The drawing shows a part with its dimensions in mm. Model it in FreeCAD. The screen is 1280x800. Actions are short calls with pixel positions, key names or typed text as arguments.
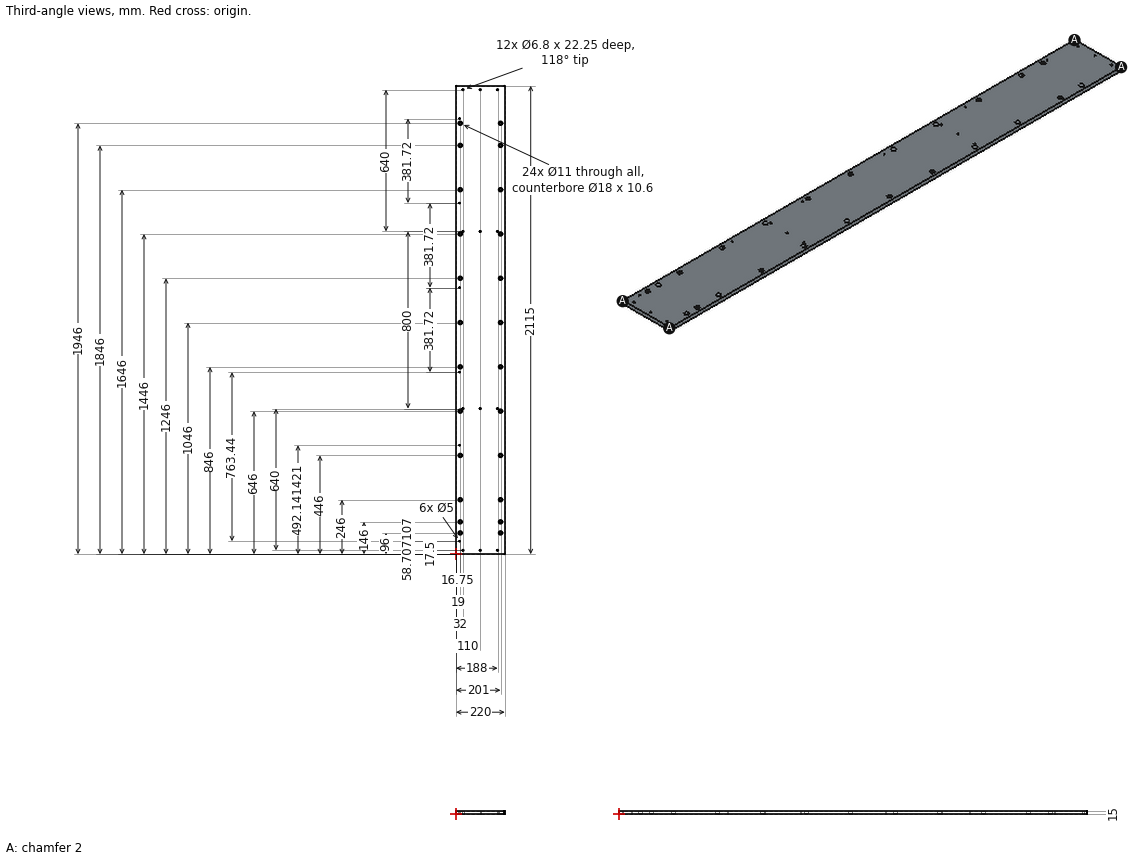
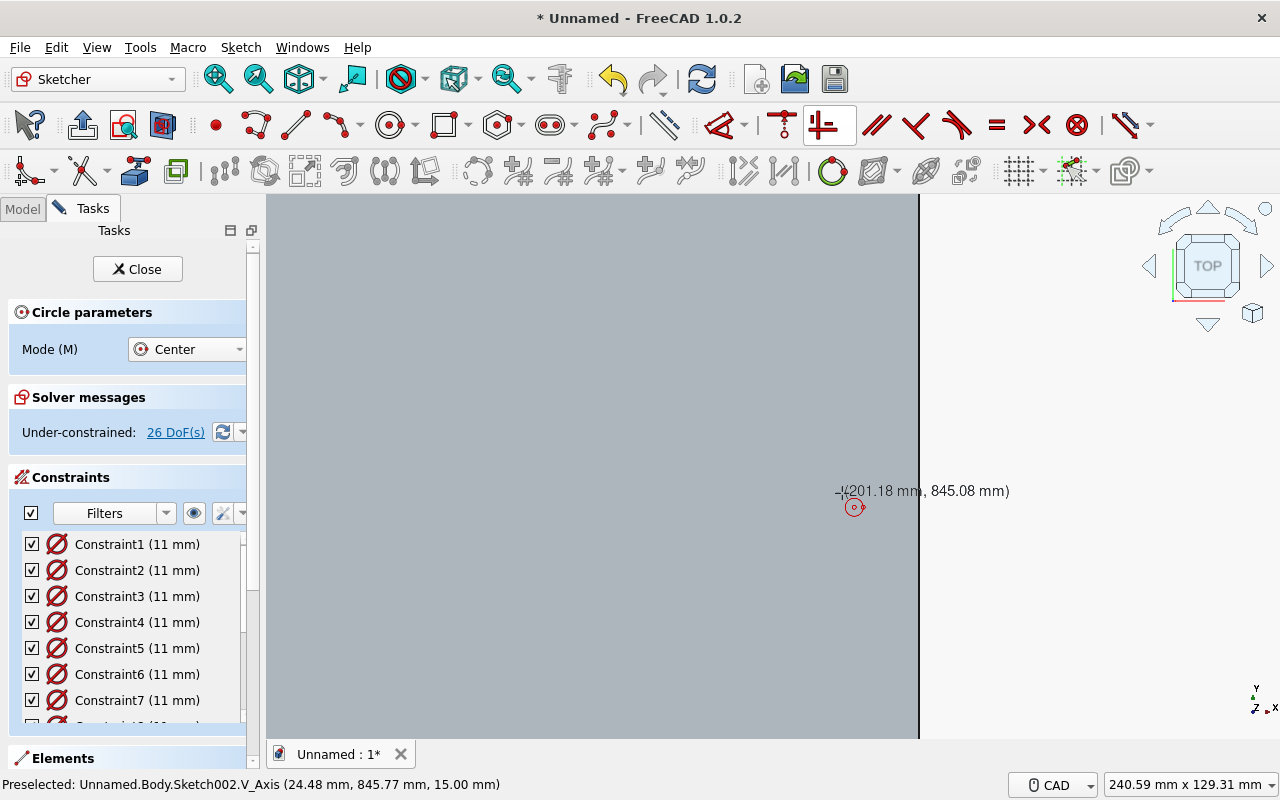
scroll(719, 494, down, 15)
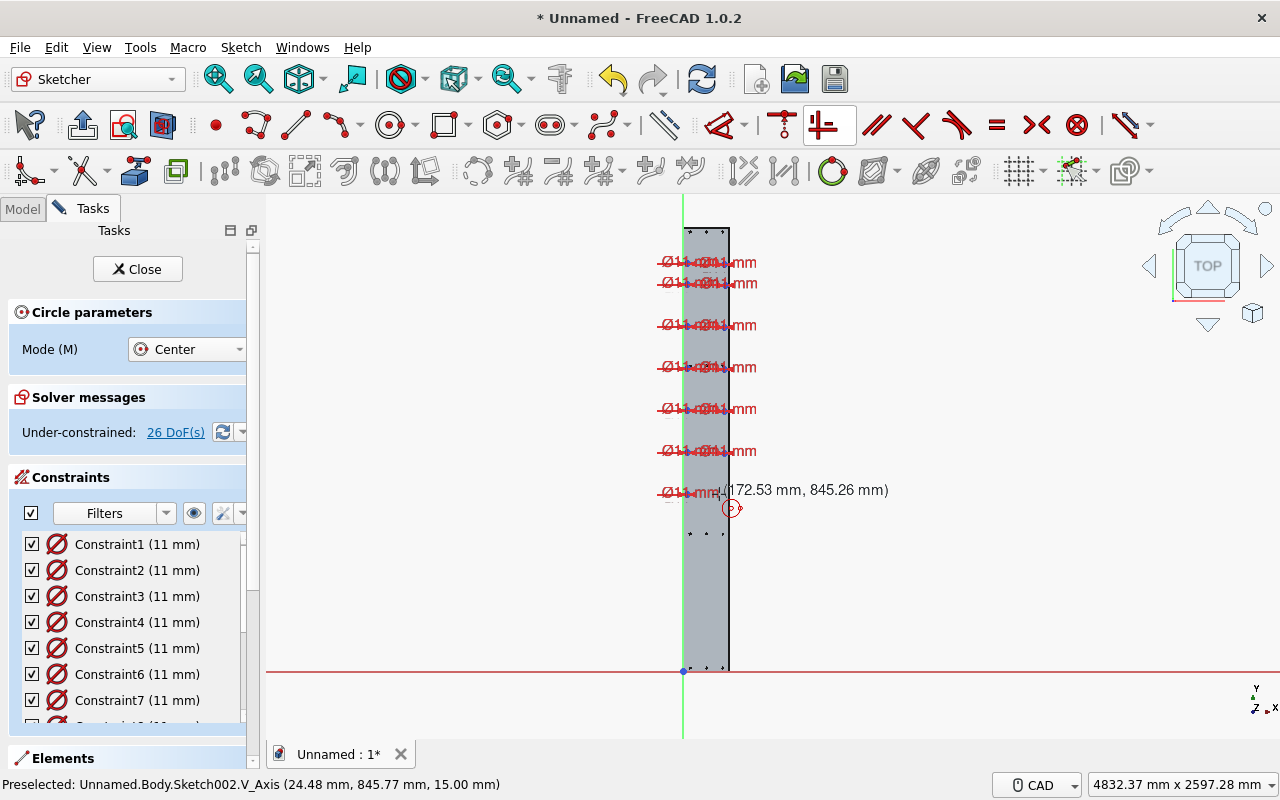
click(725, 494)
move(726, 494)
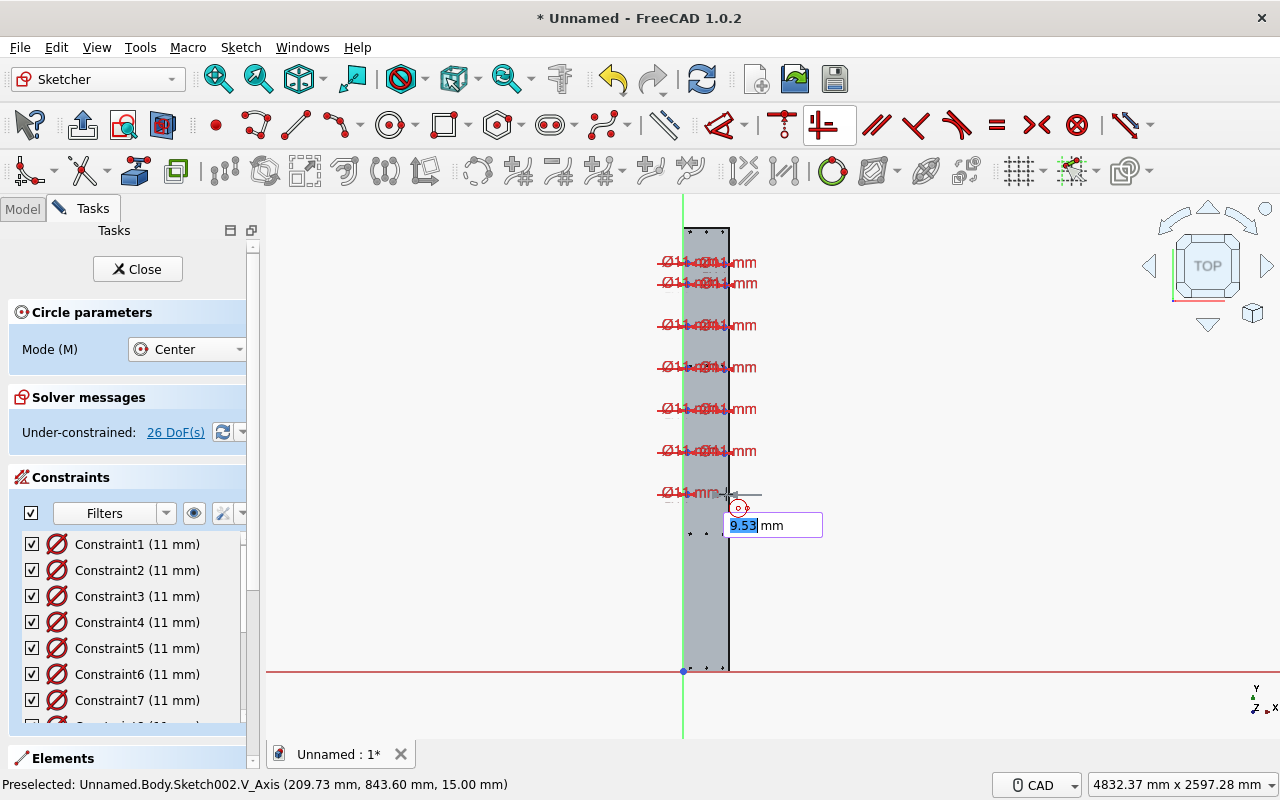
text(11)
key(Return)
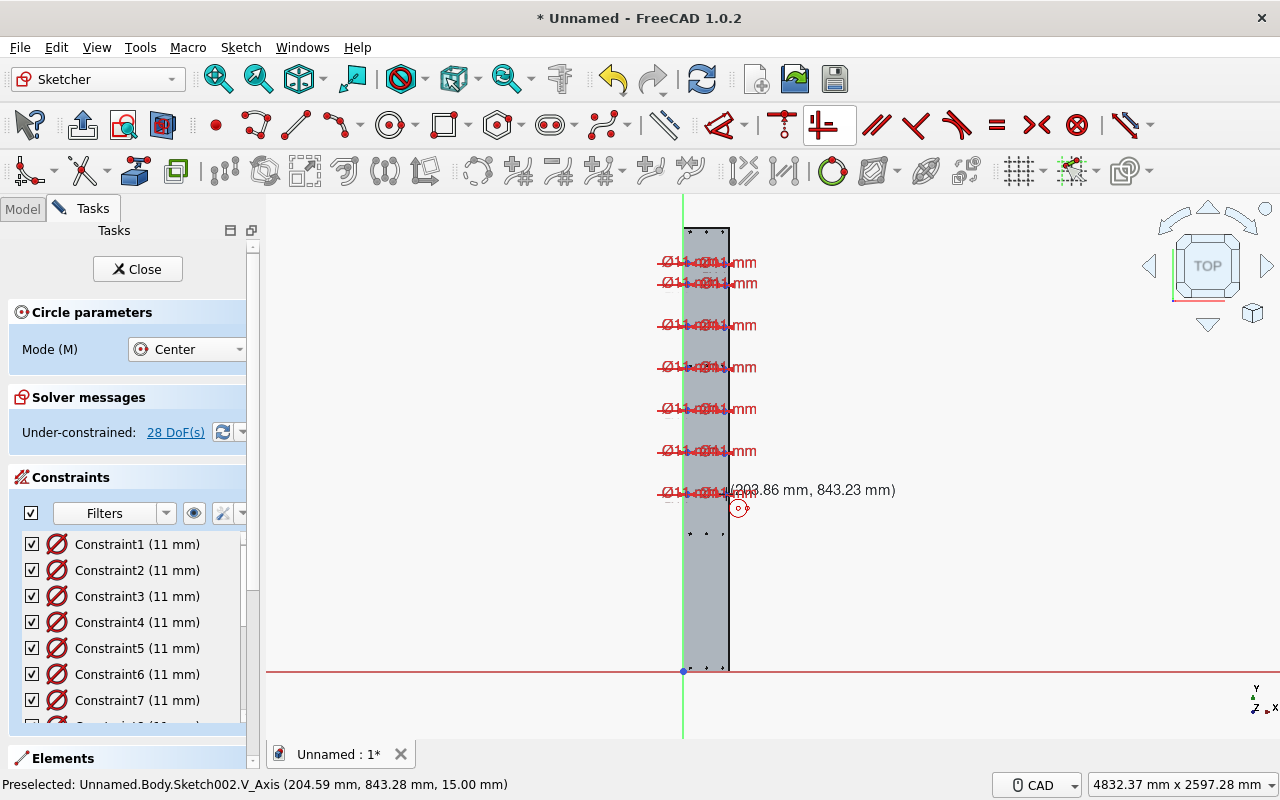
scroll(687, 536, up, 15)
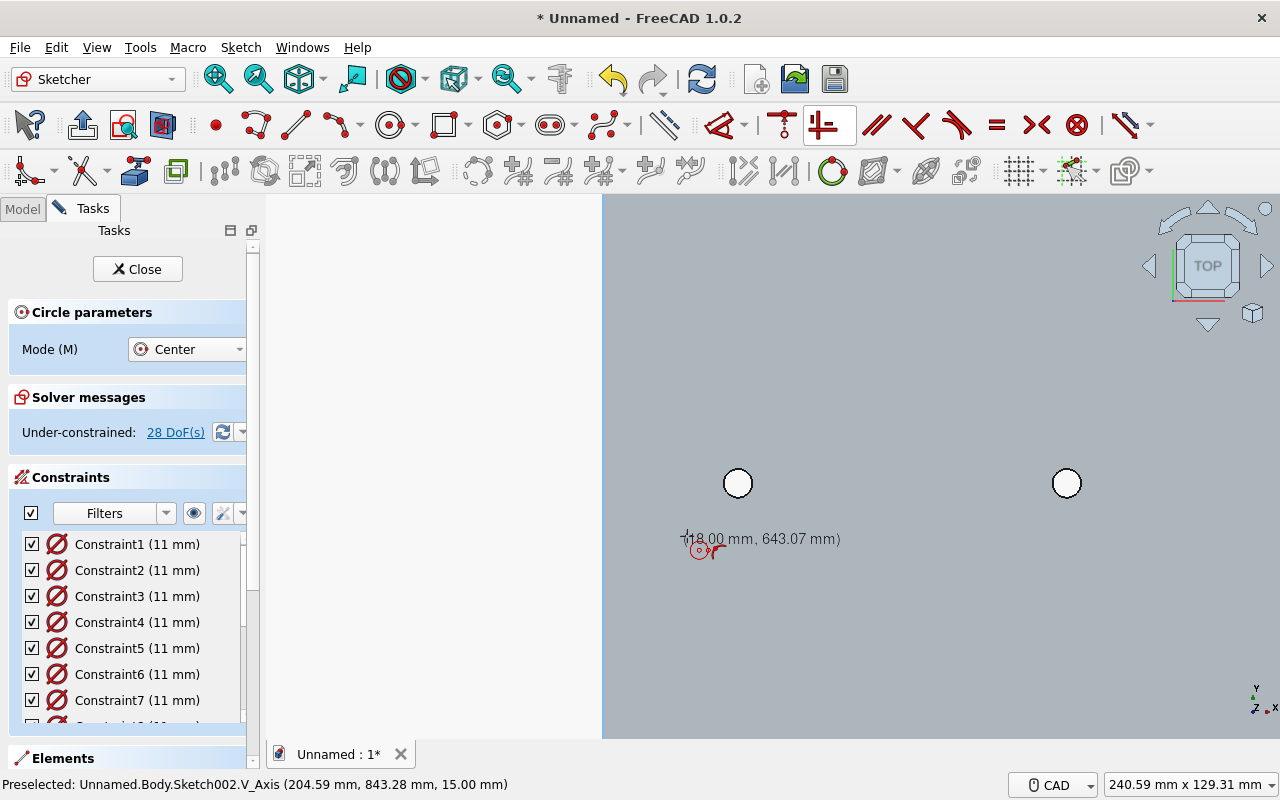
scroll(687, 536, down, 15)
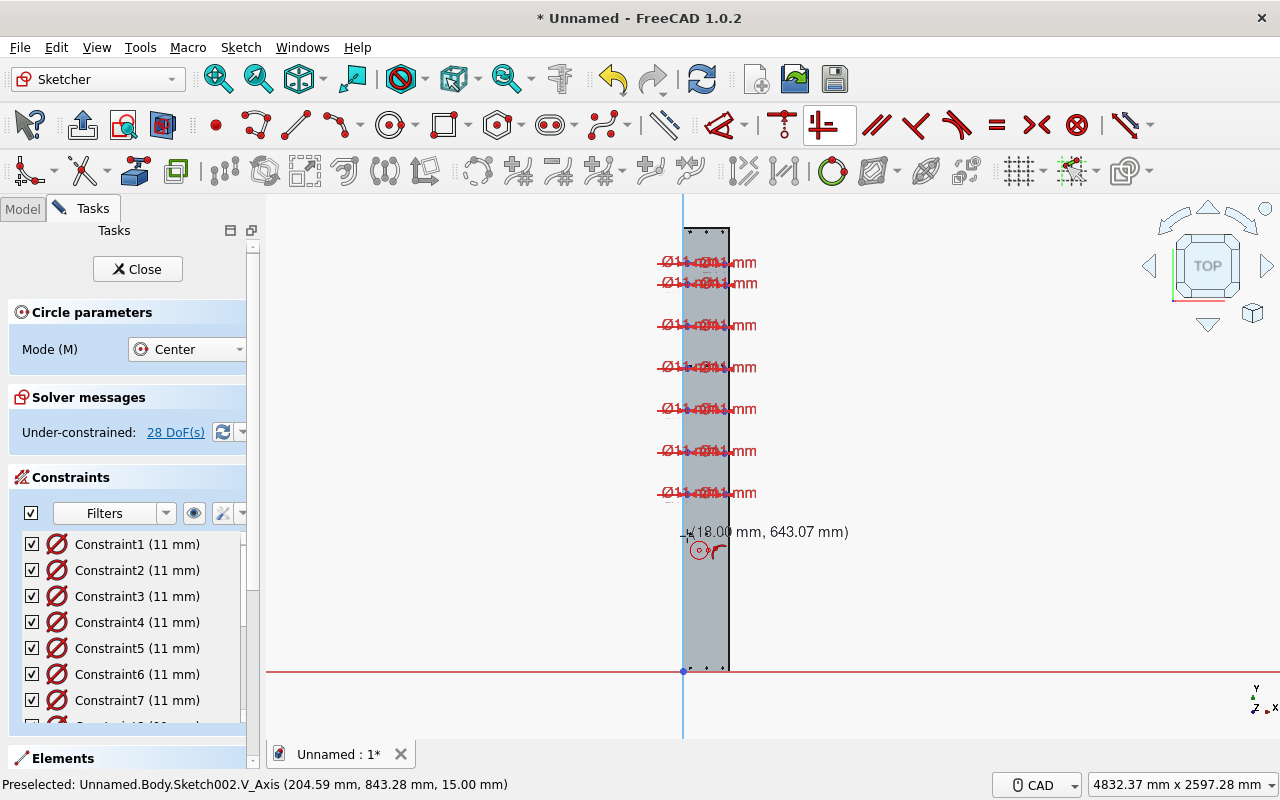
scroll(687, 536, up, 7)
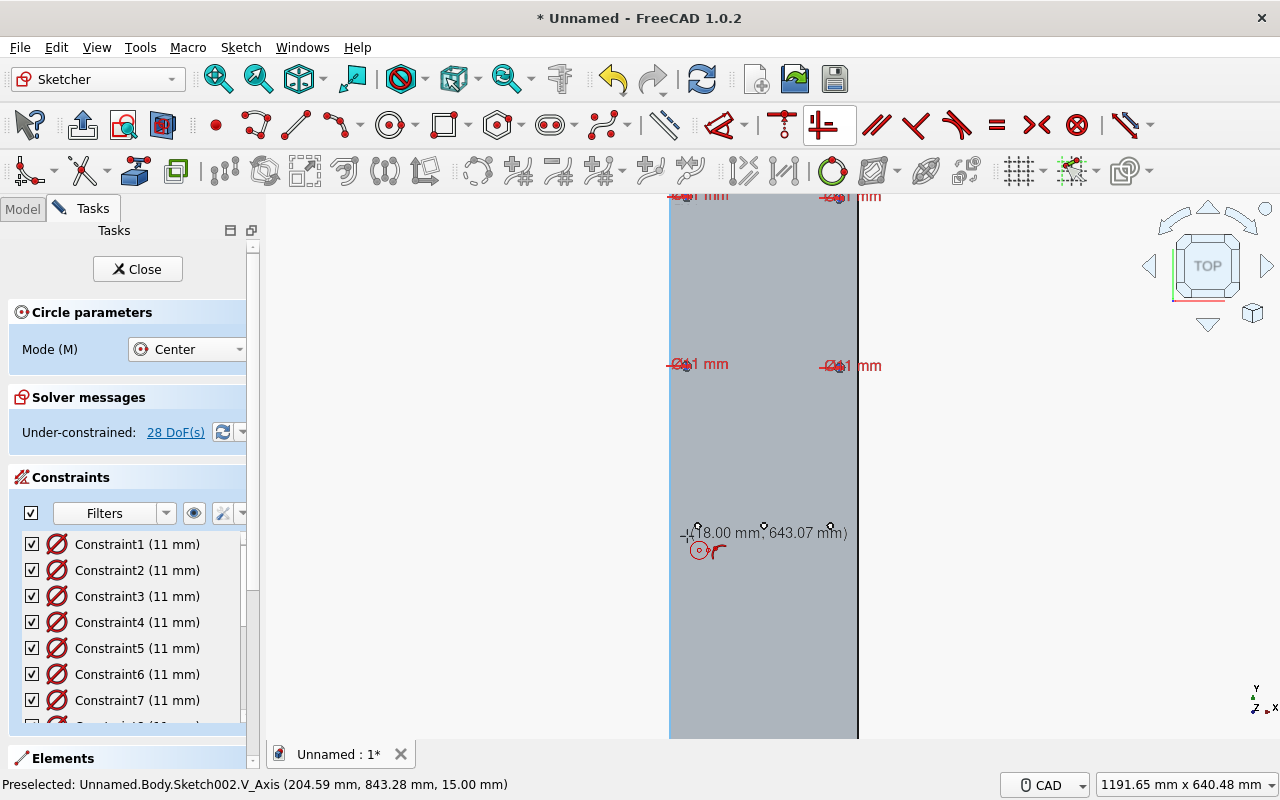
click(687, 536)
move(690, 532)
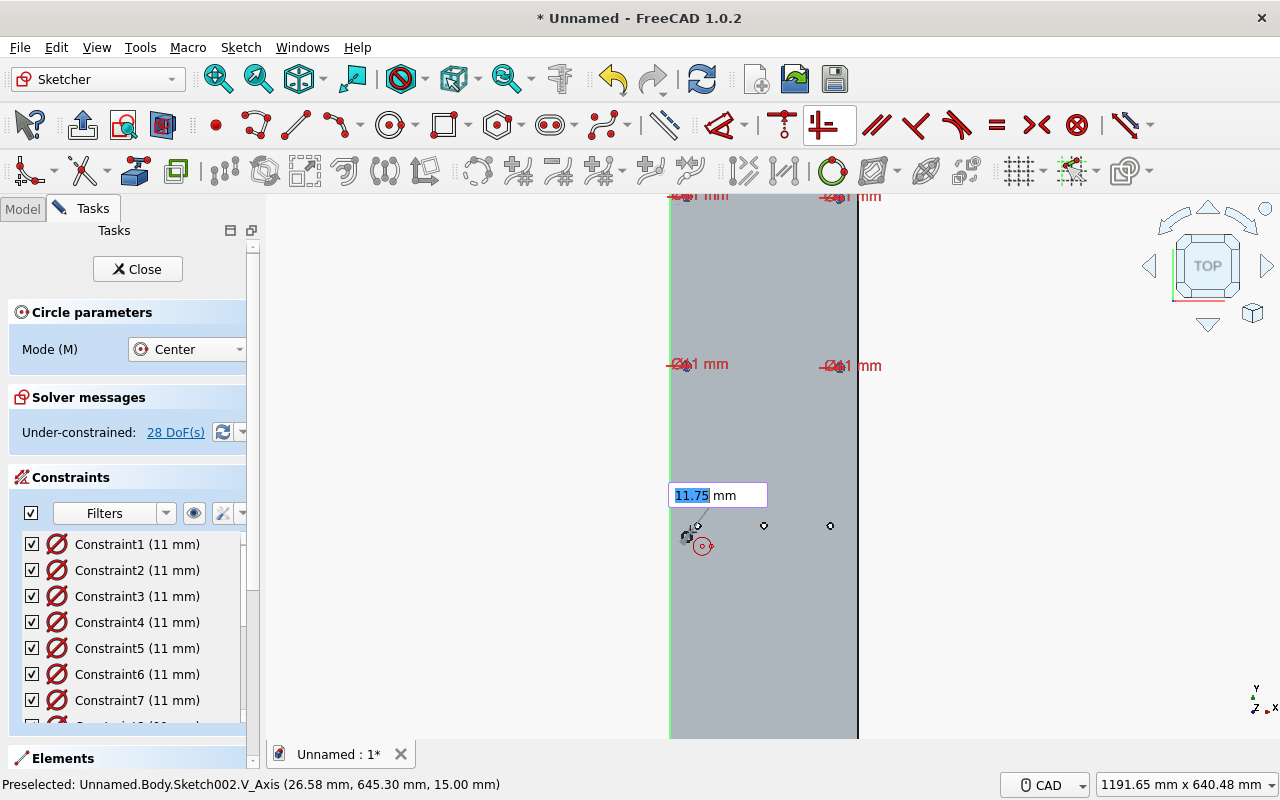
text(11)
key(Return)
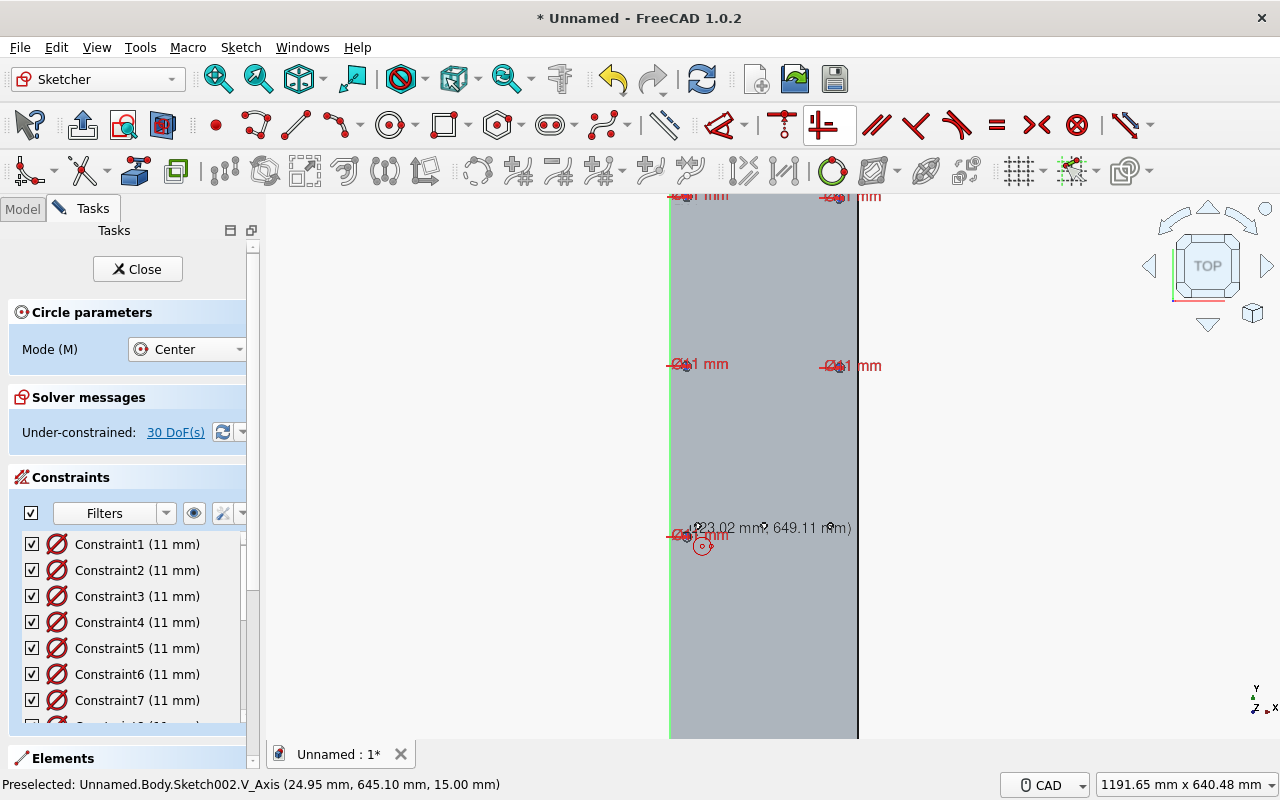
scroll(841, 536, up, 8)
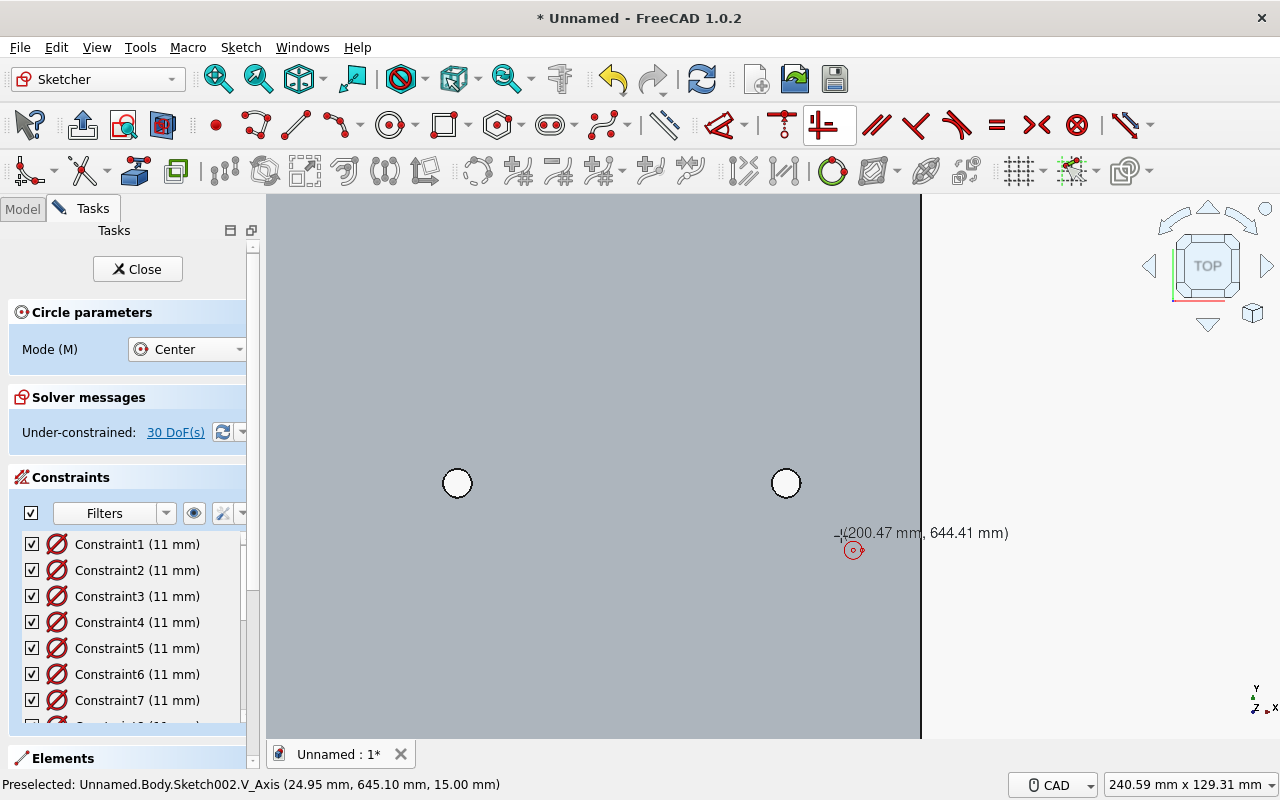
scroll(719, 536, down, 15)